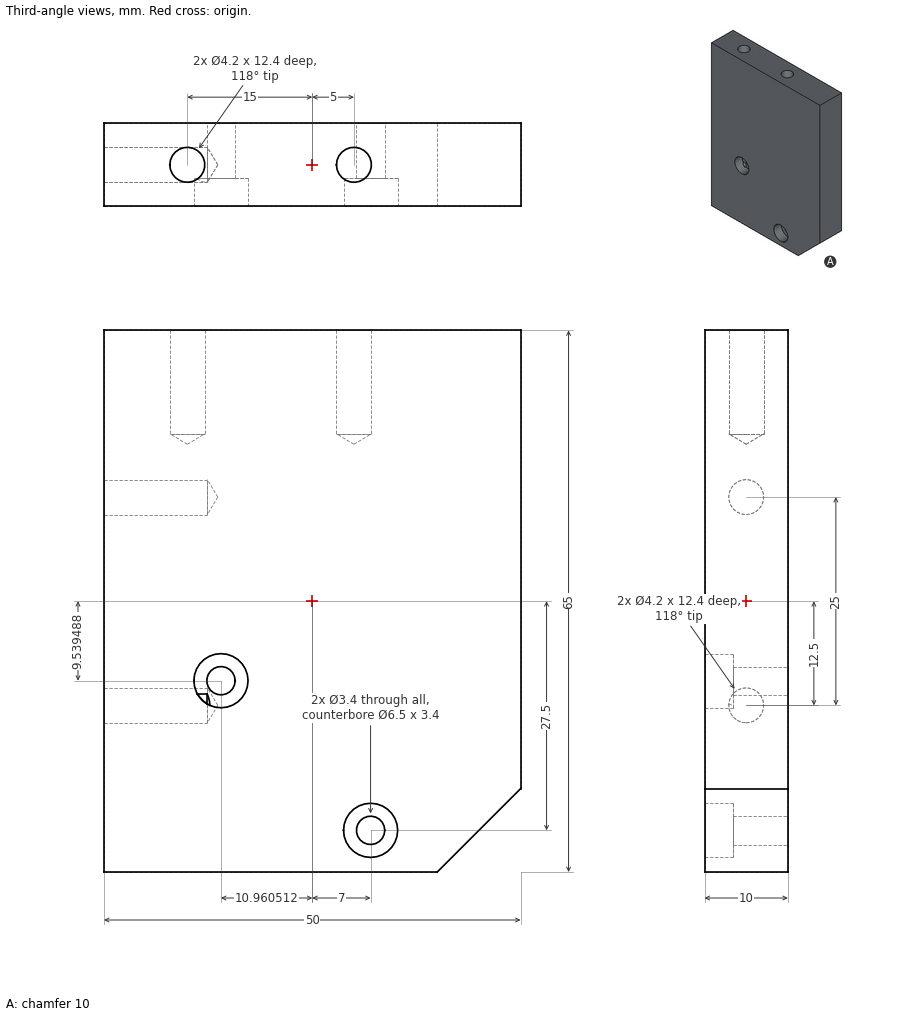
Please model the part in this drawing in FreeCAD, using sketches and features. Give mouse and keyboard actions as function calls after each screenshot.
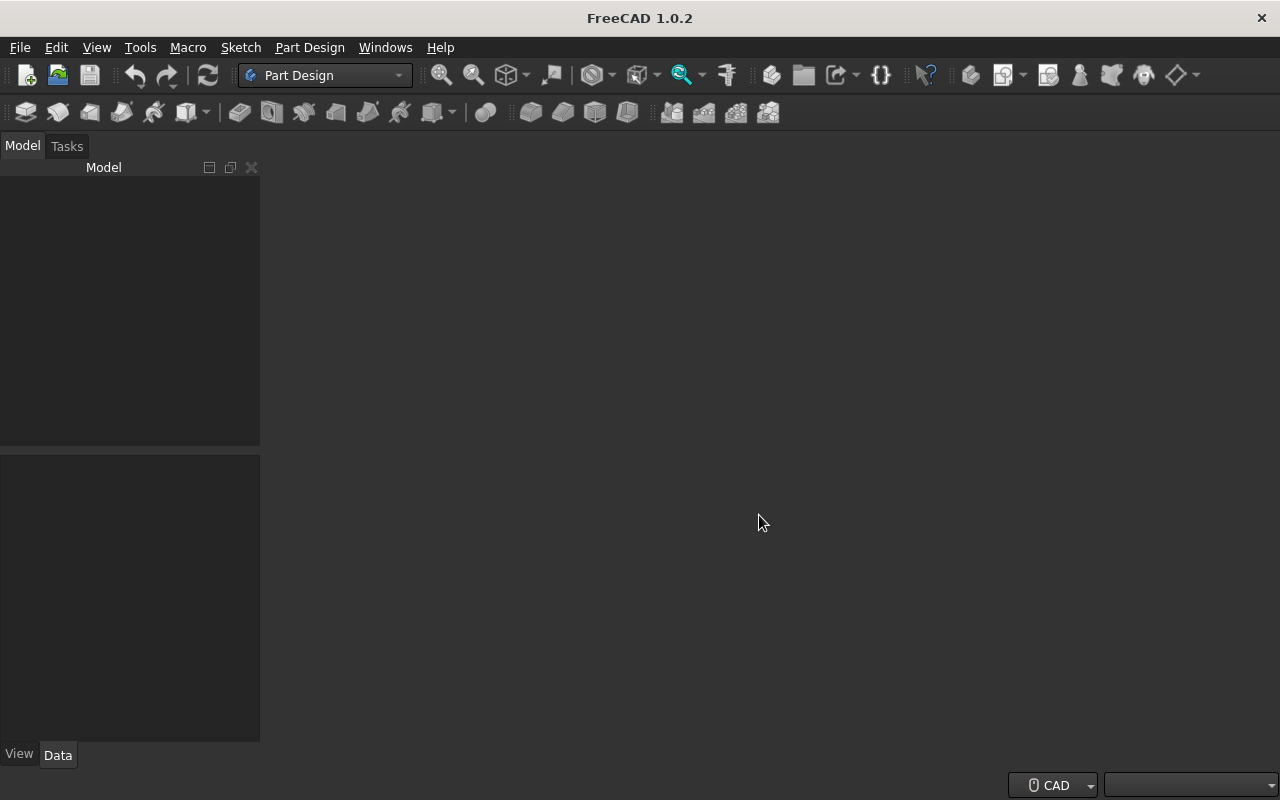
key(ctrl+n)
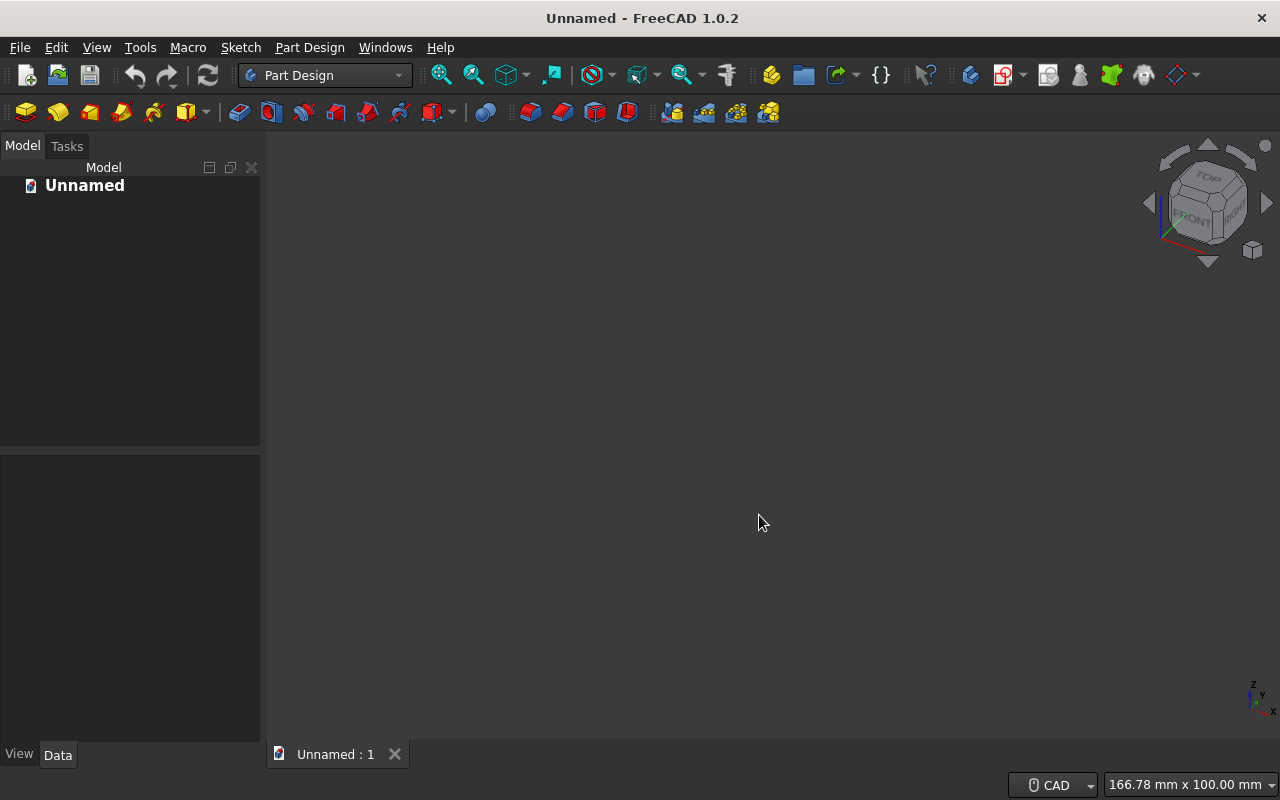
click(1004, 76)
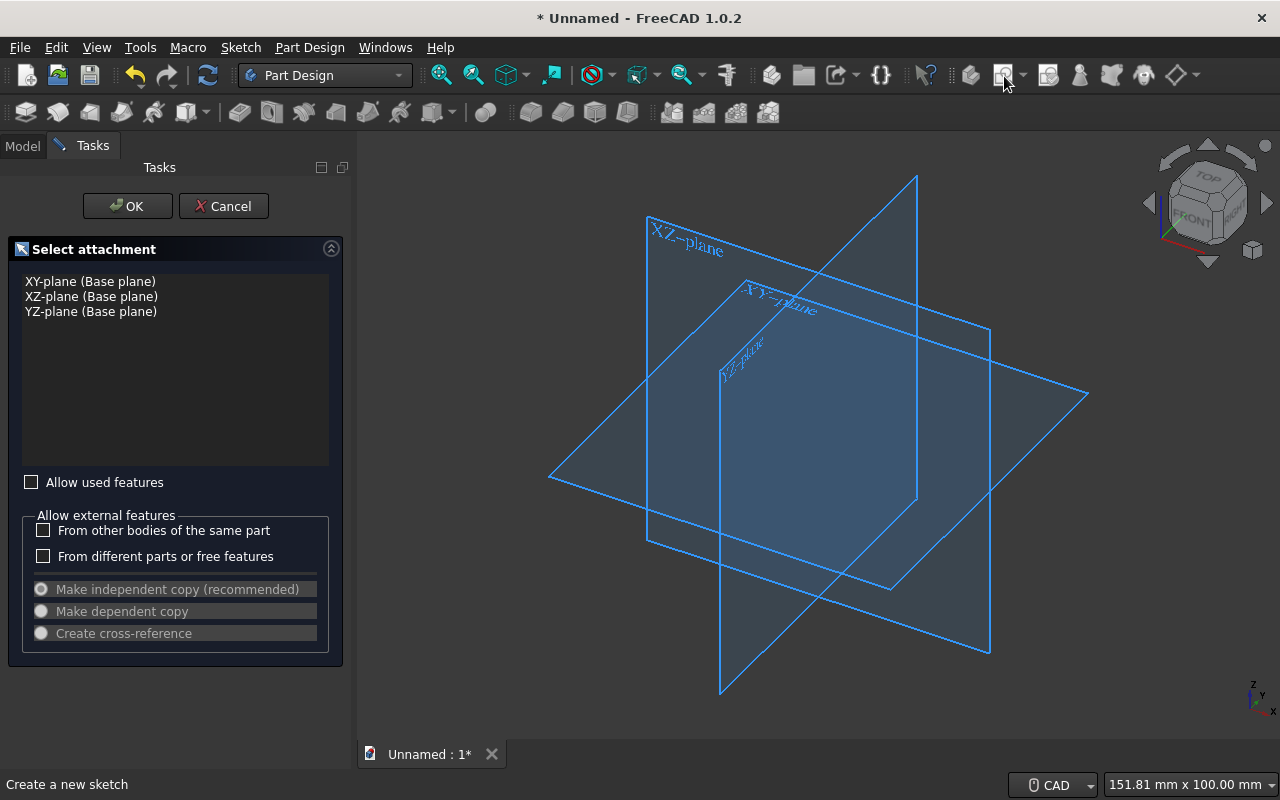
click(82, 296)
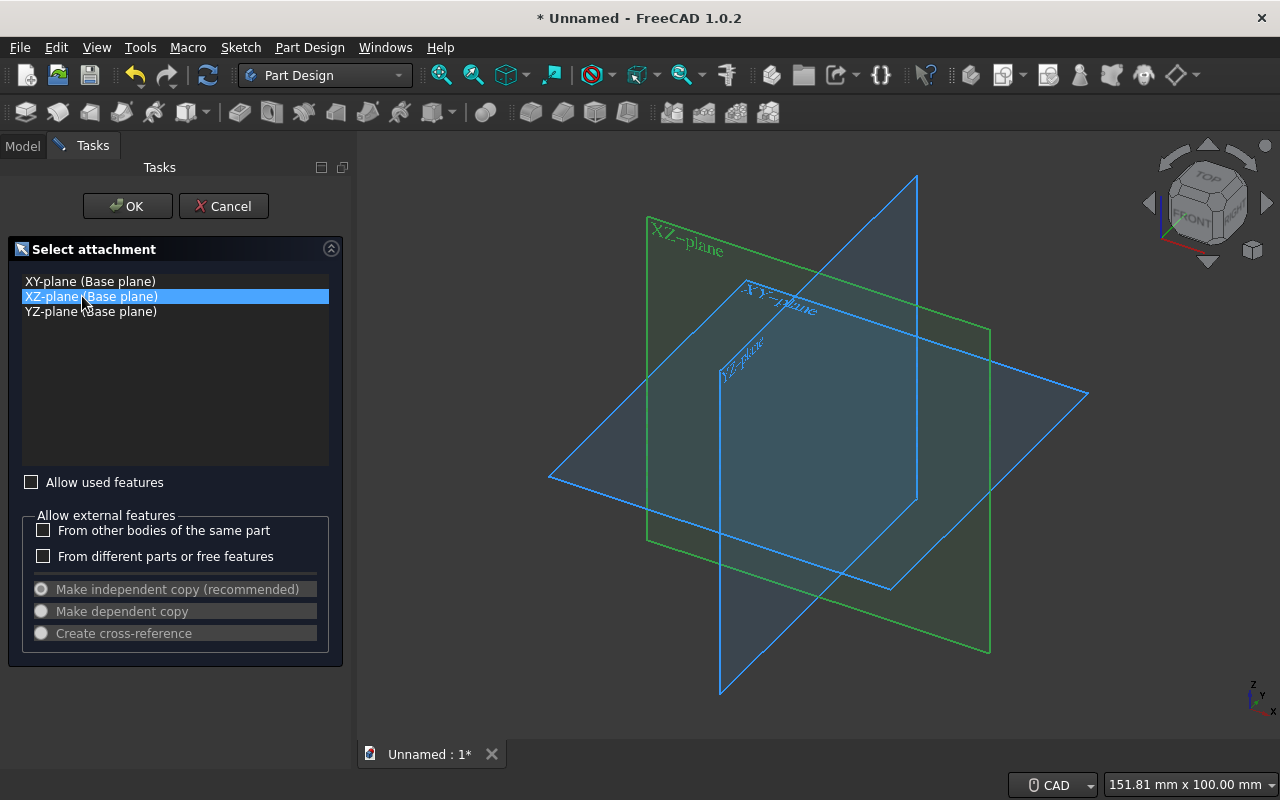
click(128, 206)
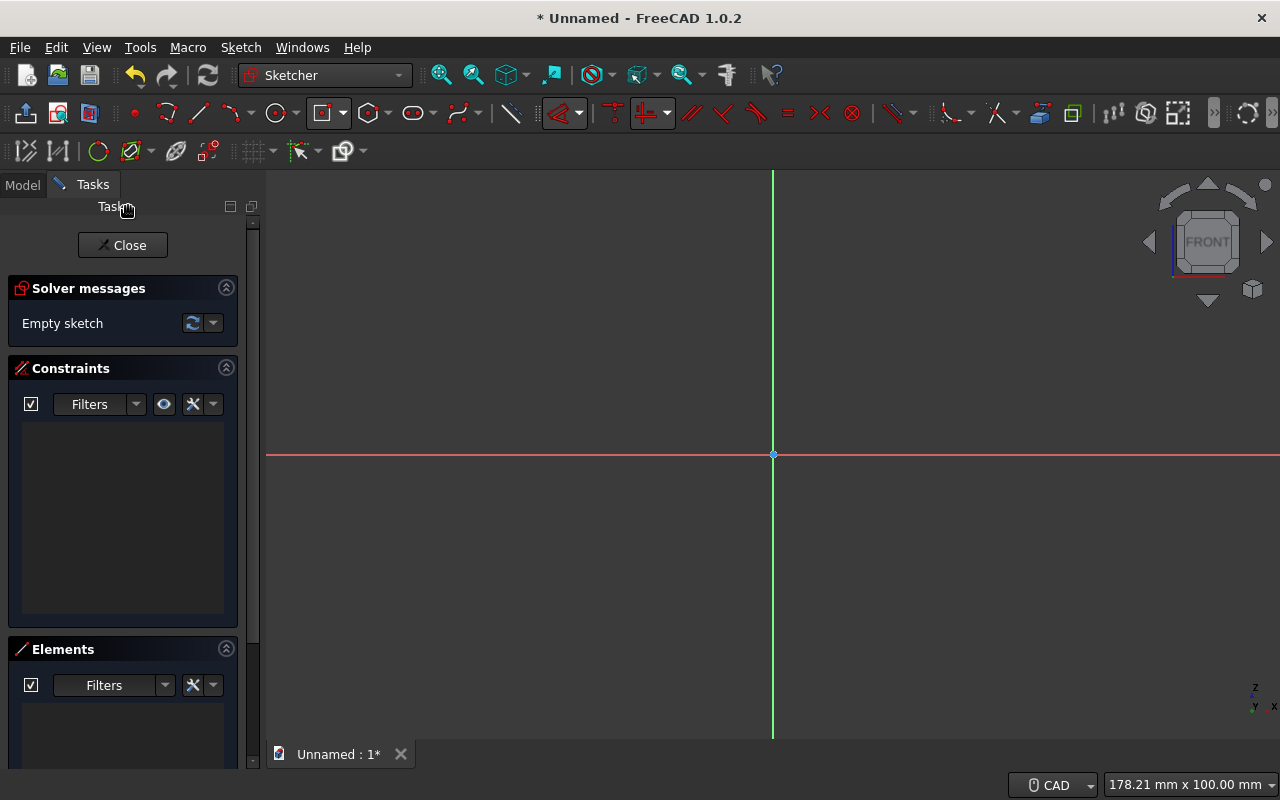
click(322, 114)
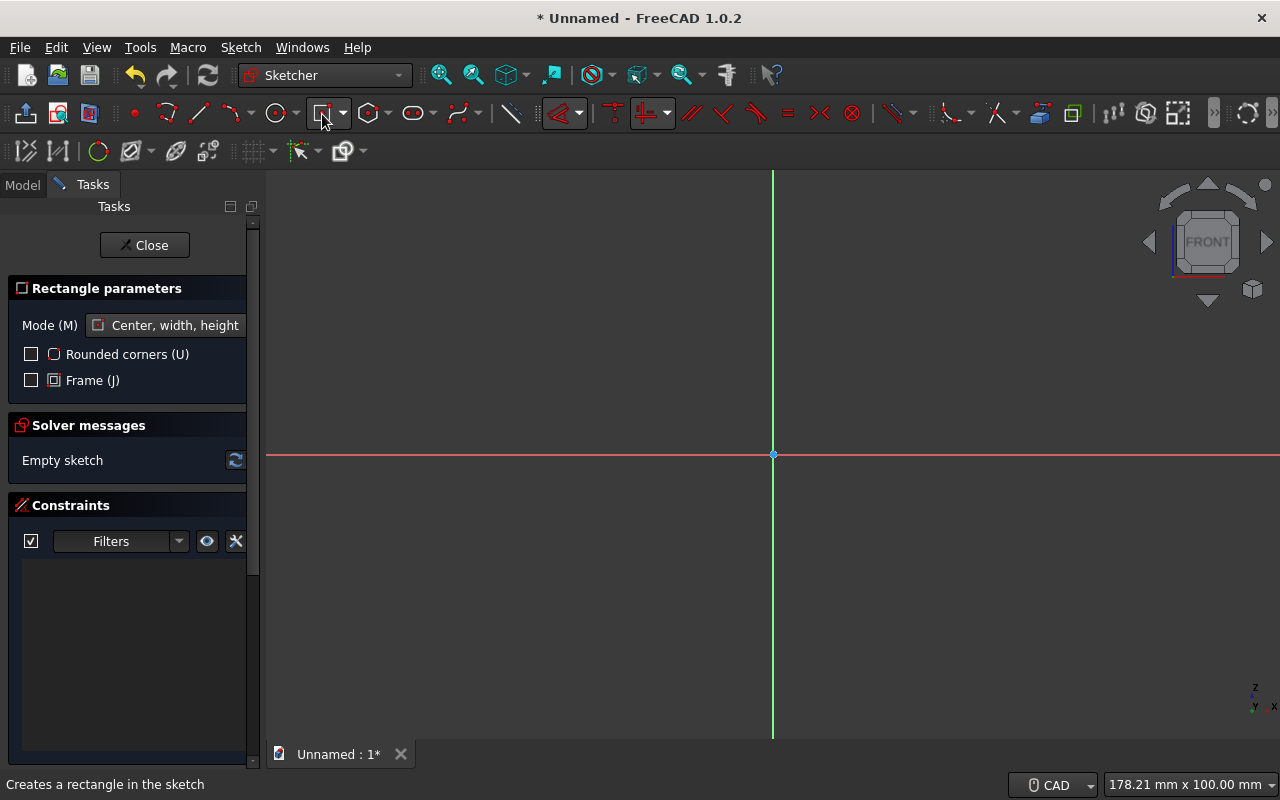
click(773, 454)
move(915, 270)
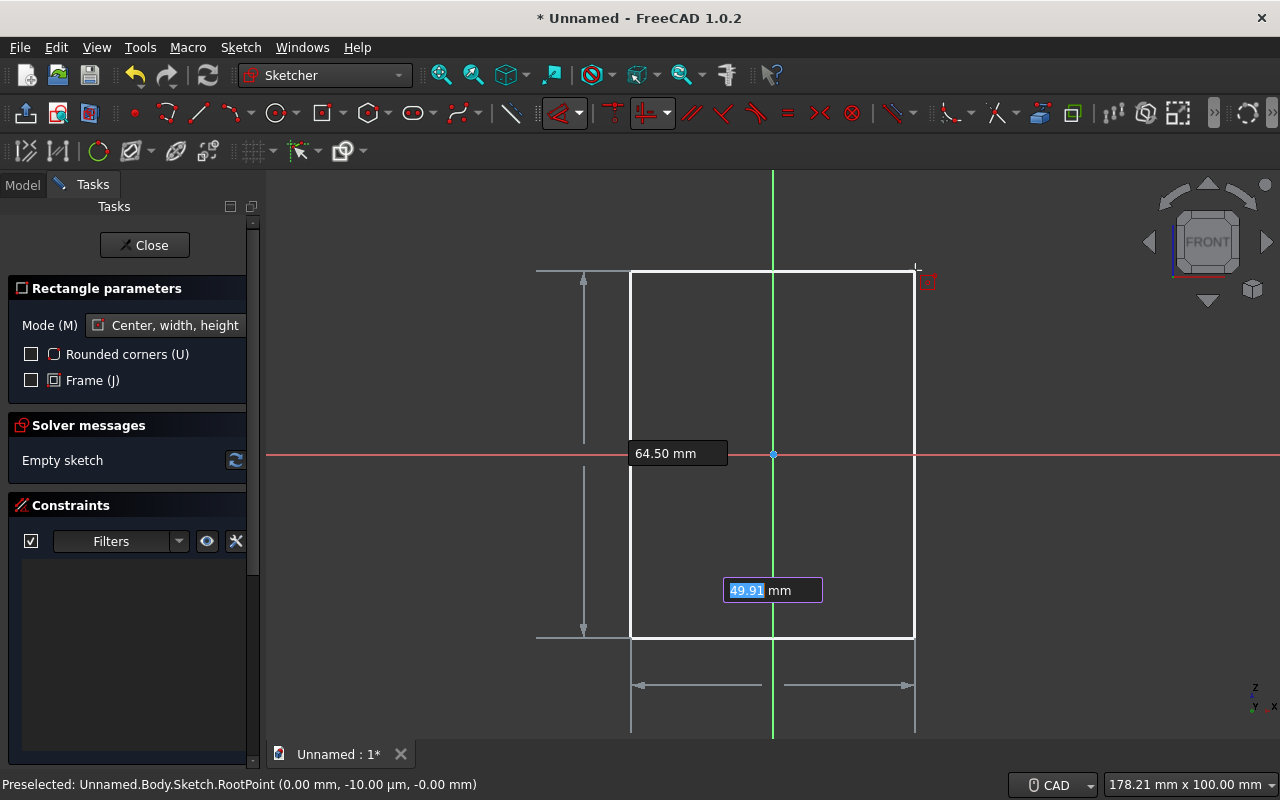
text(50)
key(Tab)
text(65)
key(Return)
key(Escape)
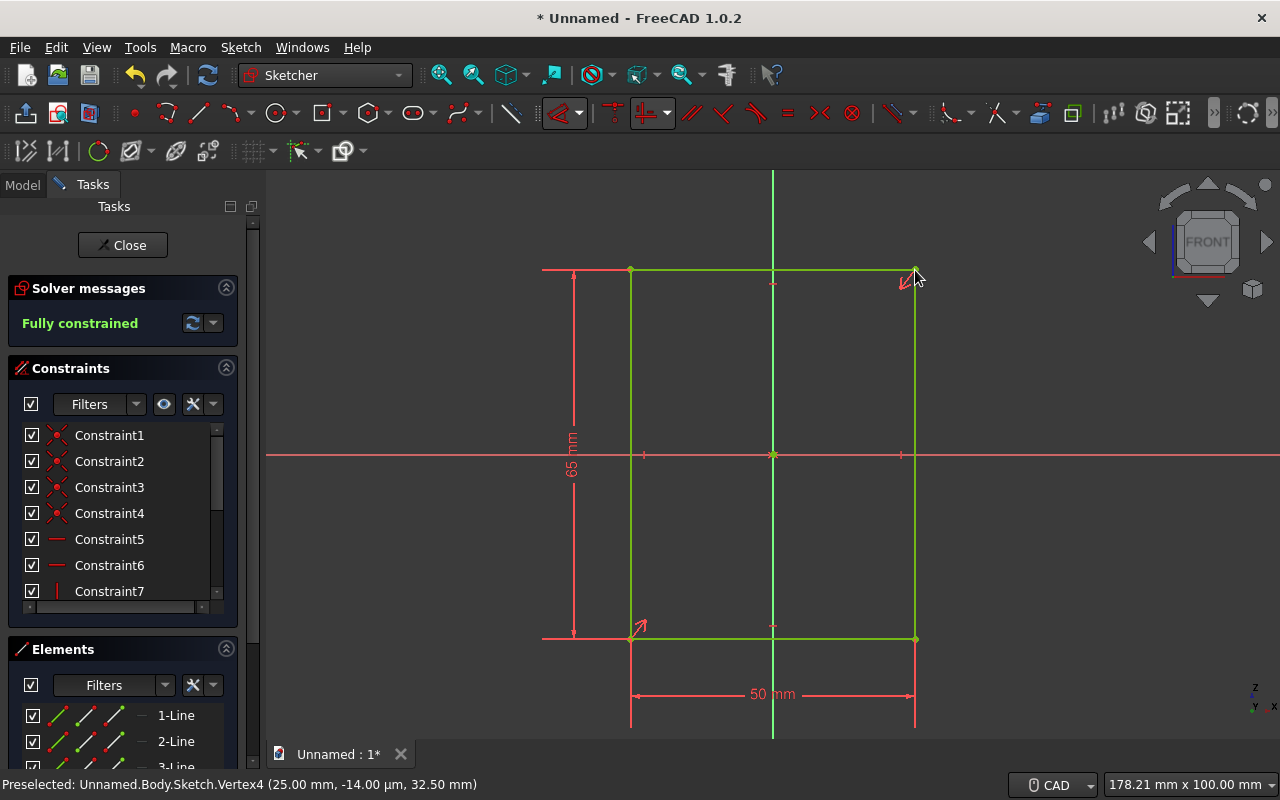
click(123, 245)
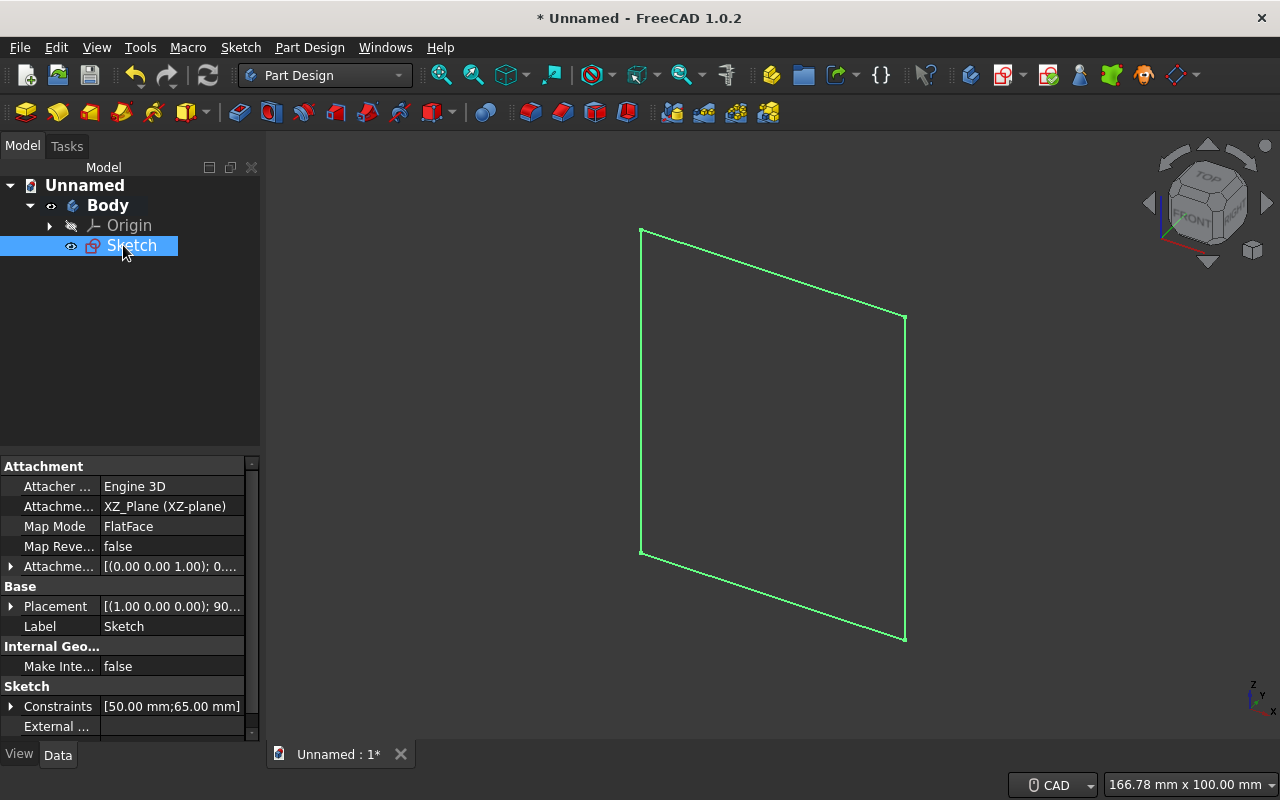
click(26, 112)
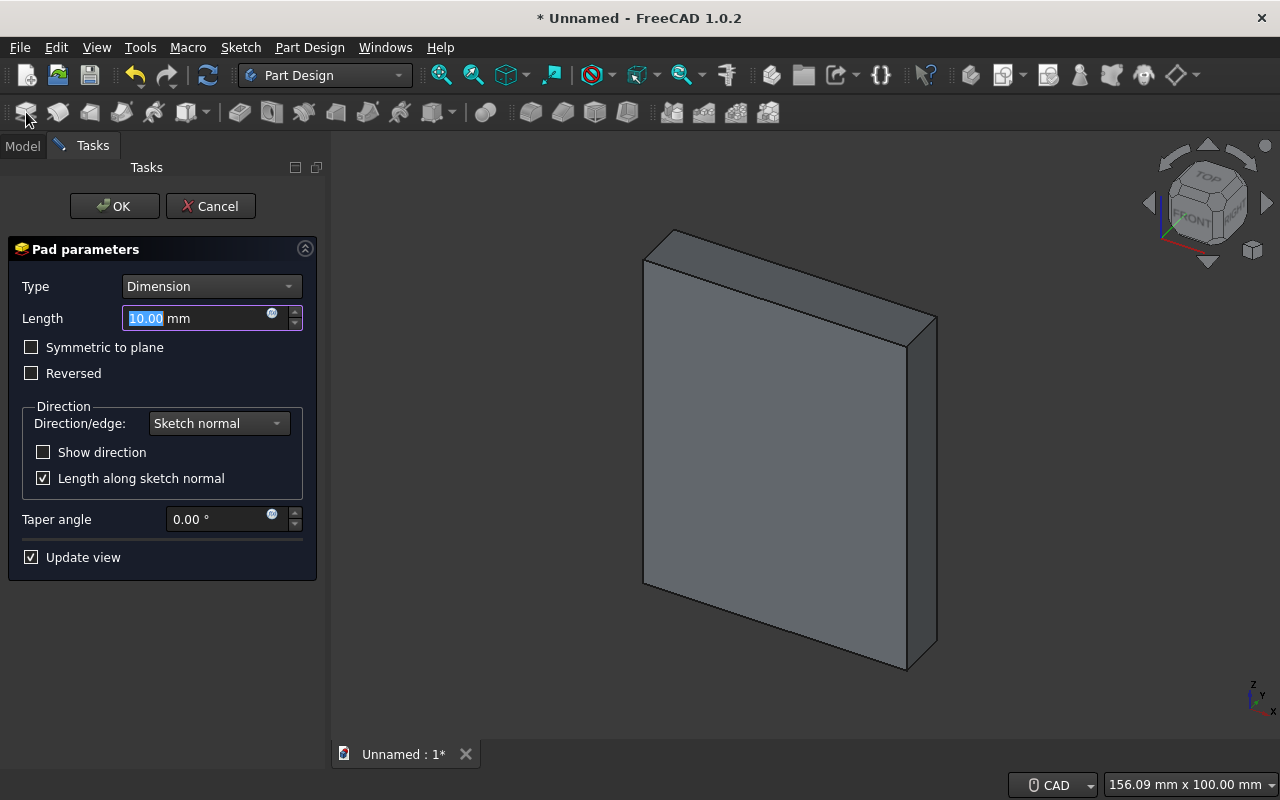
text(10)
key(Tab)